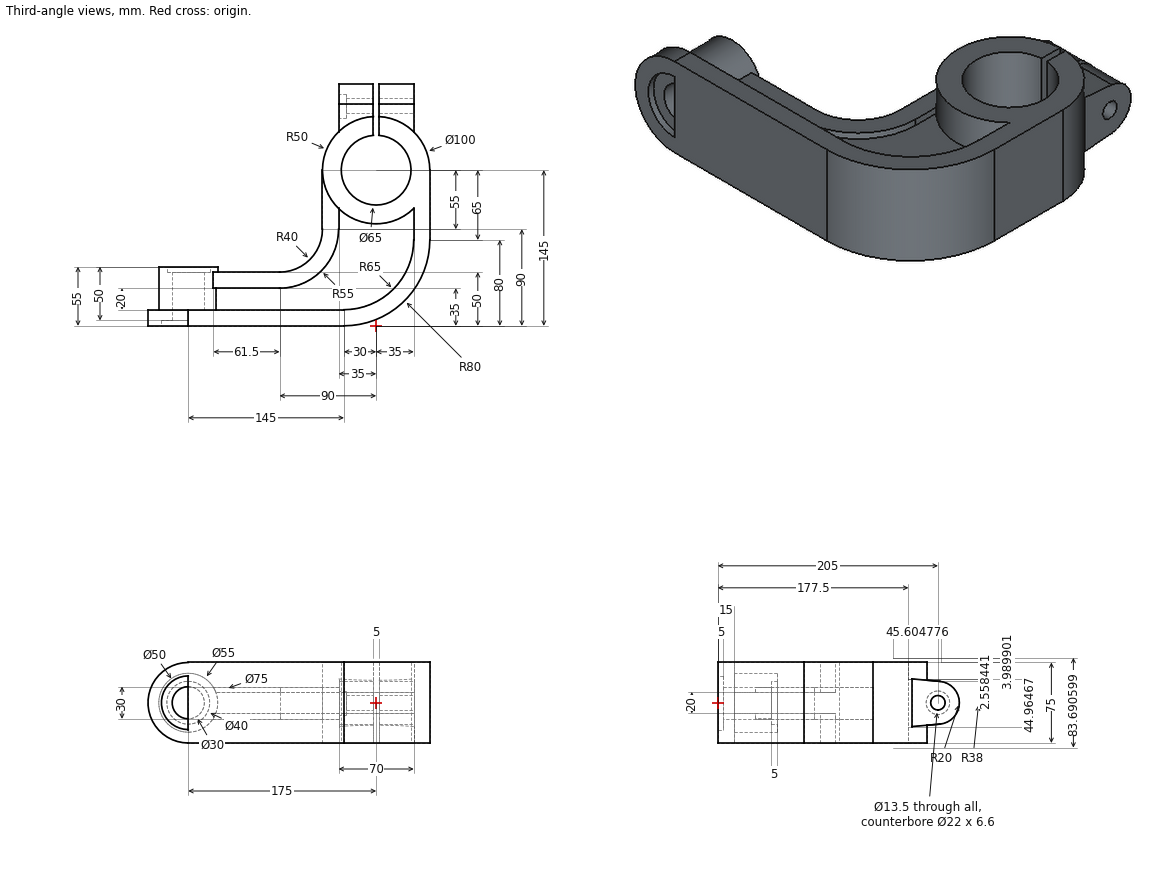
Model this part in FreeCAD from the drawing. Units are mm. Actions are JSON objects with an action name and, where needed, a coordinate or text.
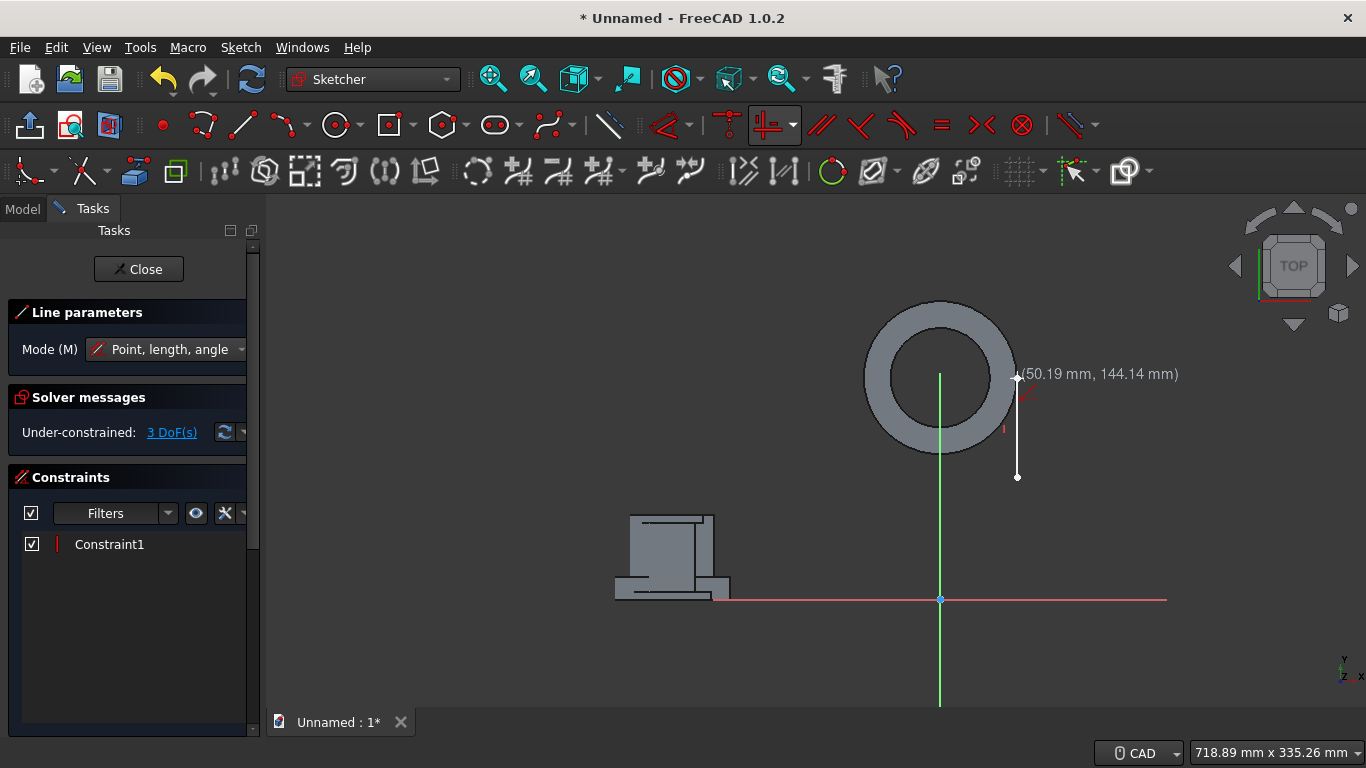
{"action": "left_click", "coordinate": [994, 432]}
{"action": "left_click", "coordinate": [994, 477]}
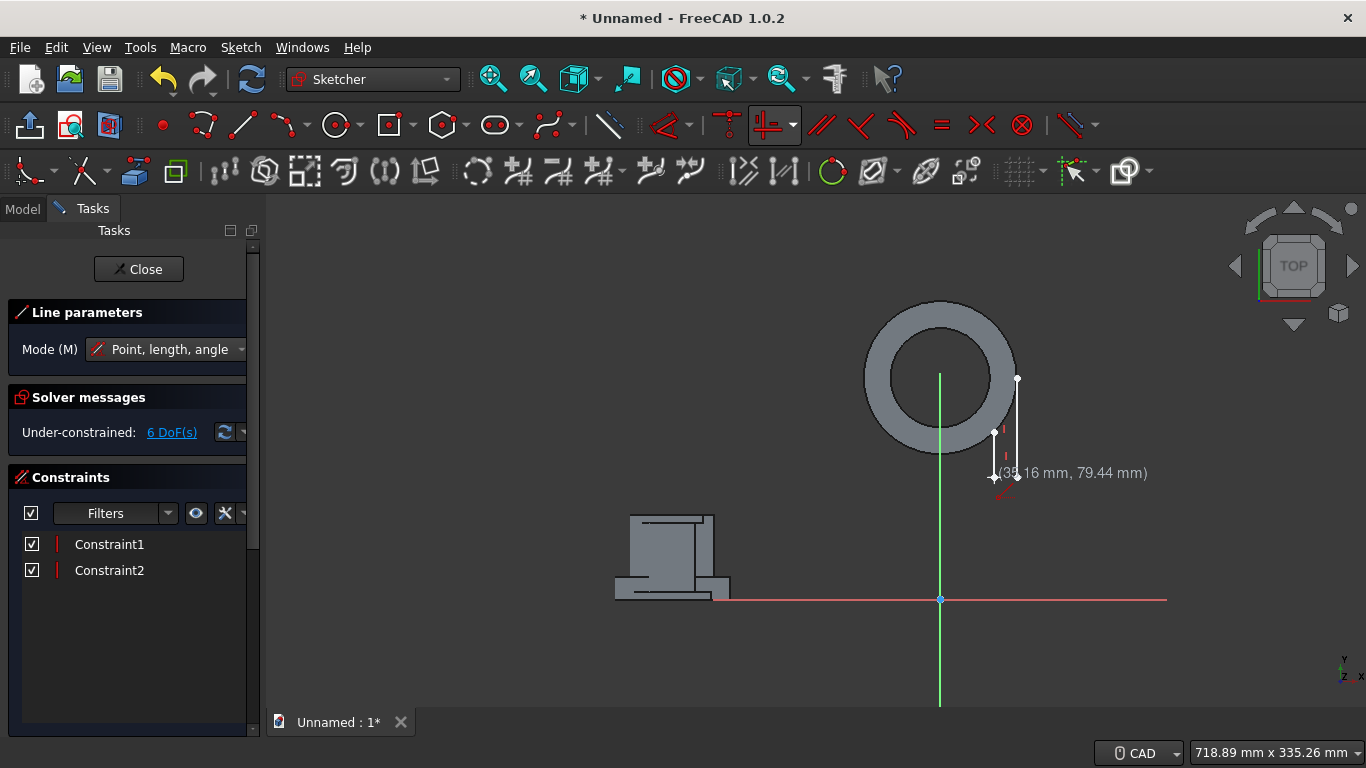
{"action": "key", "text": "g m"}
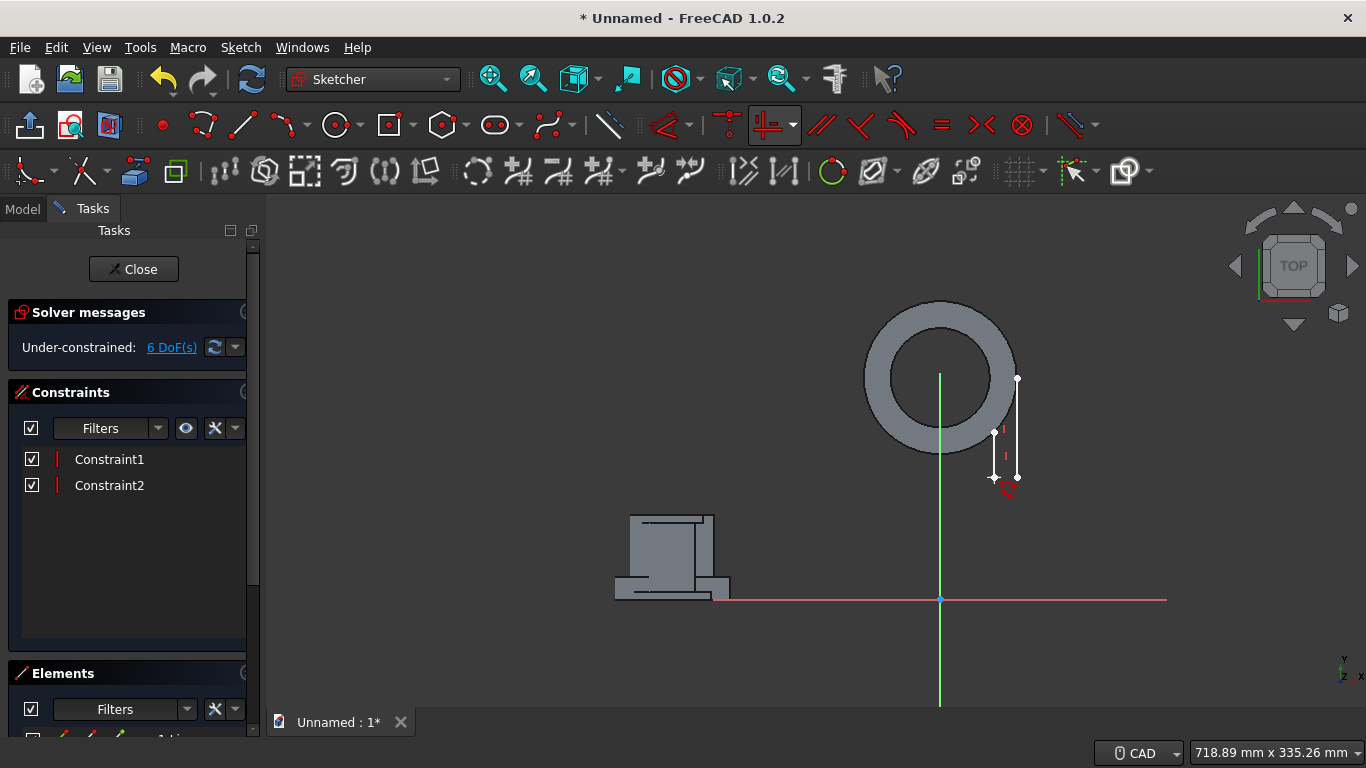
{"action": "left_click", "coordinate": [894, 577]}
{"action": "left_click", "coordinate": [672, 577]}
{"action": "left_click", "coordinate": [672, 600]}
{"action": "left_click", "coordinate": [894, 591]}
{"action": "right_click", "coordinate": [894, 591]}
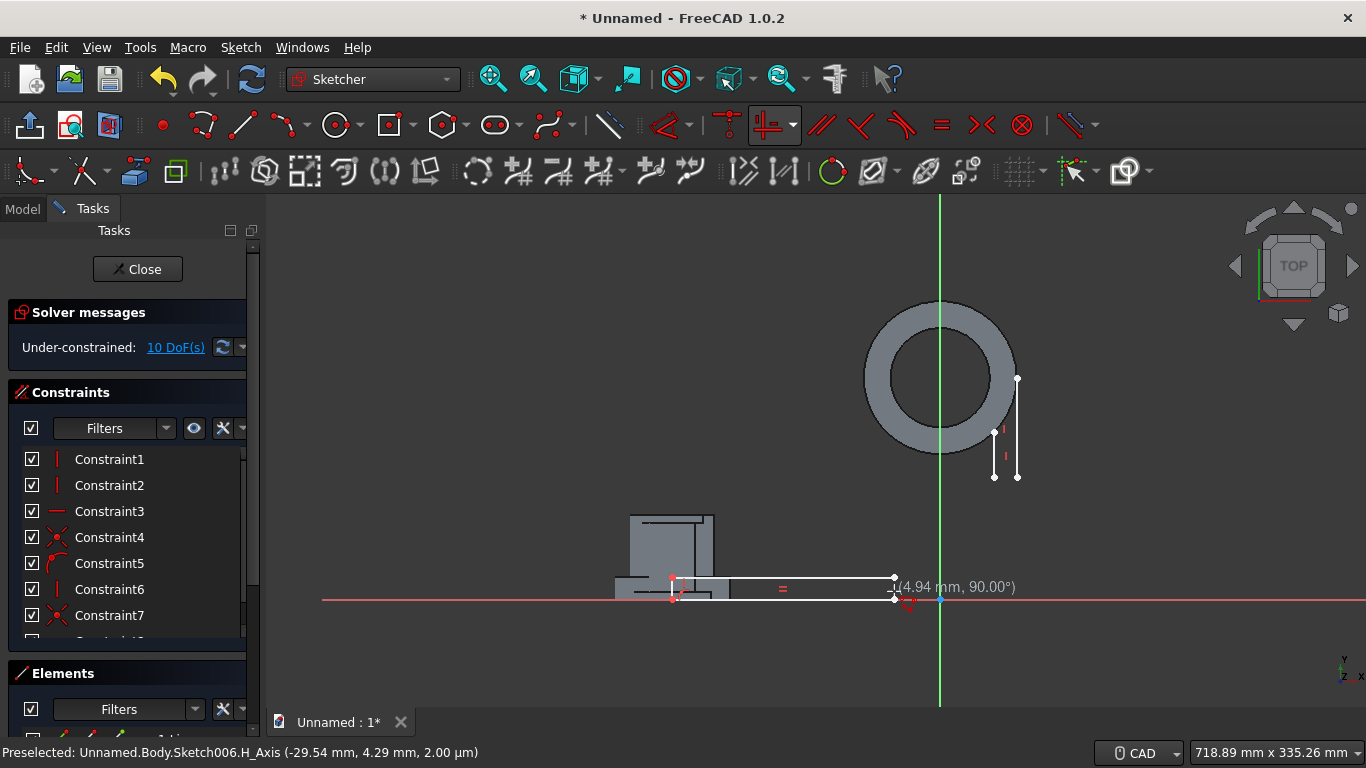
{"action": "key", "text": "g 3 a"}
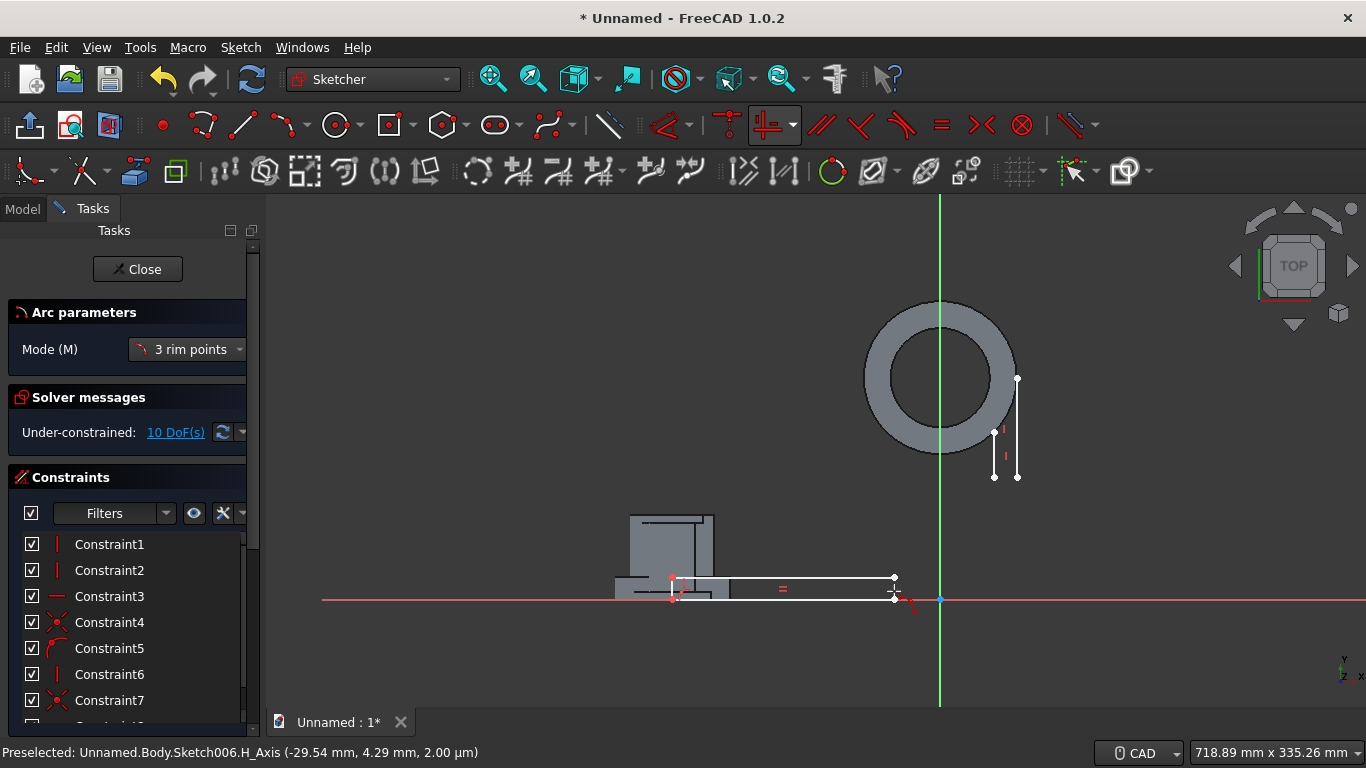
{"action": "left_click", "coordinate": [1017, 379]}
{"action": "left_click", "coordinate": [994, 433]}
{"action": "left_click", "coordinate": [870, 348]}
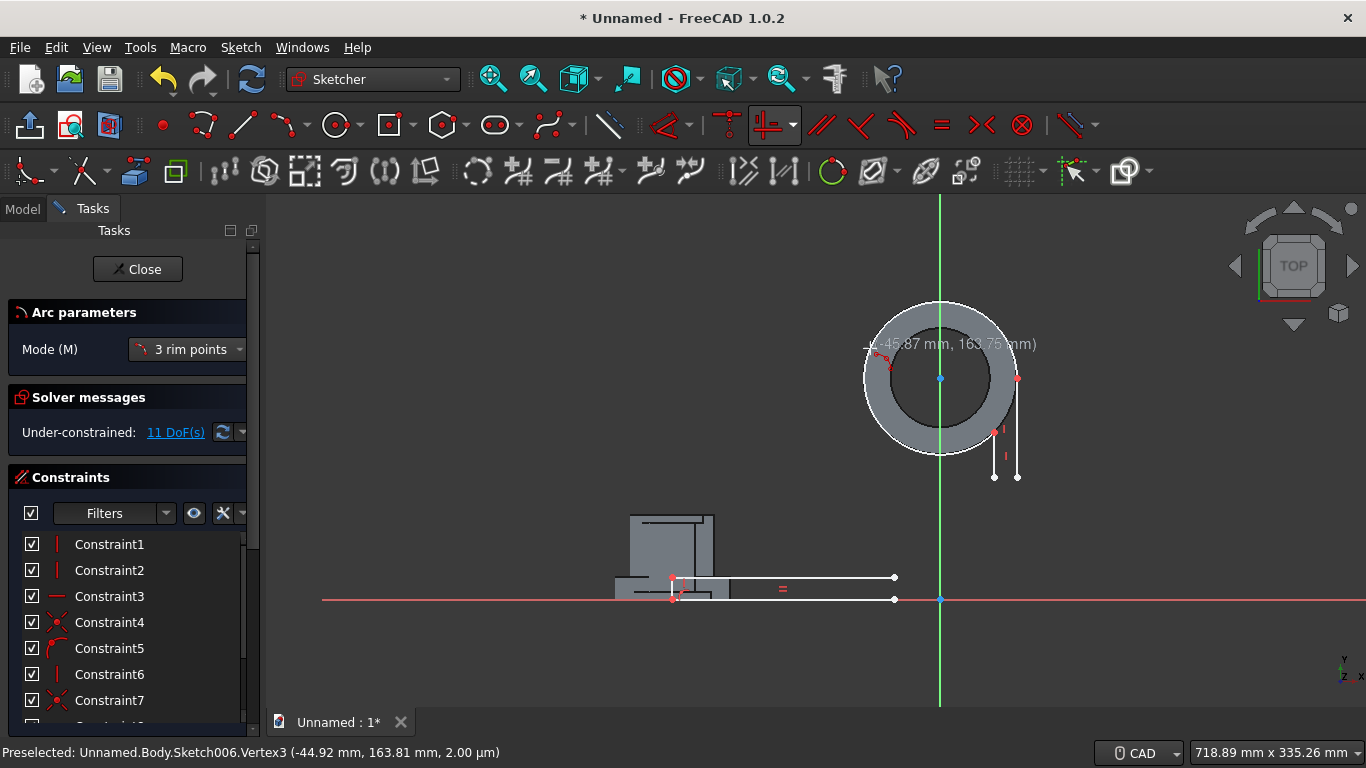
{"action": "left_click", "coordinate": [994, 478]}
{"action": "left_click", "coordinate": [894, 578]}
{"action": "left_click", "coordinate": [965, 547]}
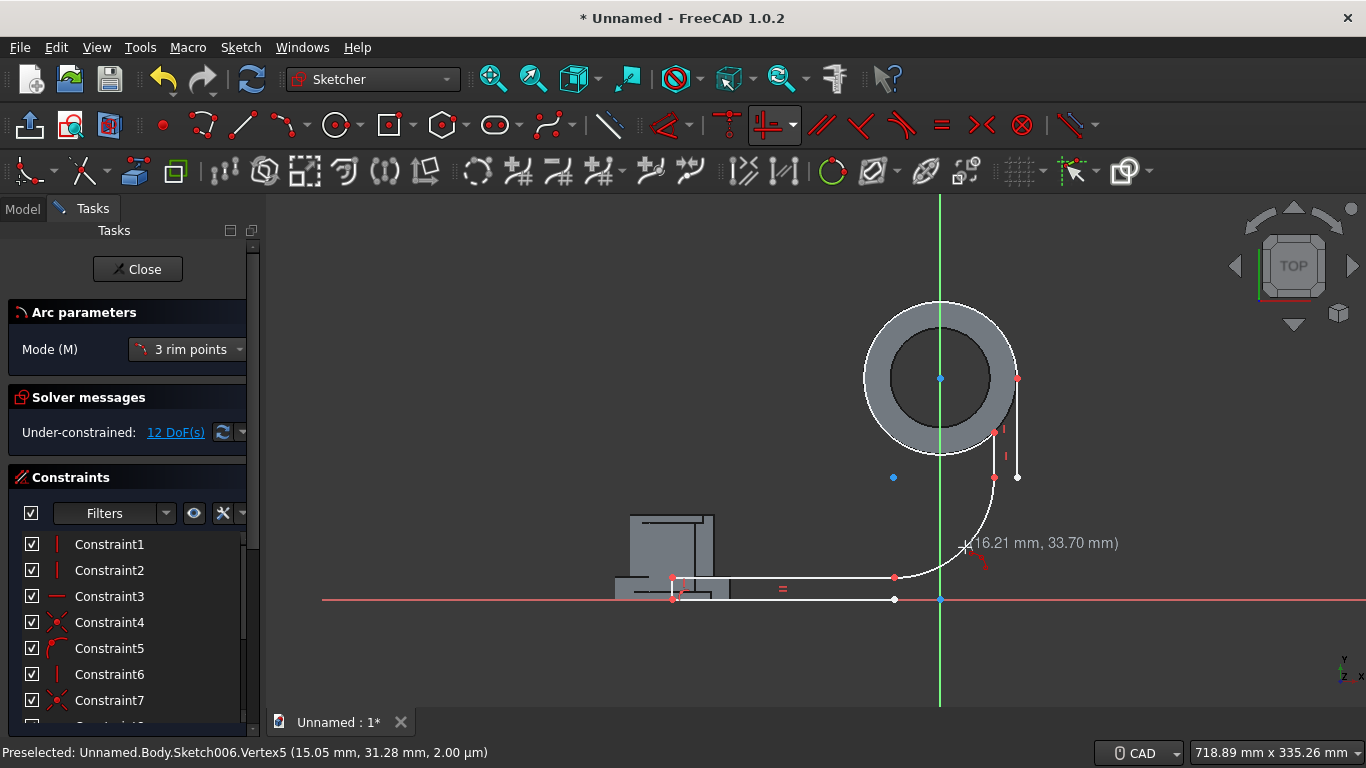
{"action": "left_click", "coordinate": [894, 600]}
{"action": "left_click", "coordinate": [1017, 478]}
{"action": "left_click", "coordinate": [981, 564]}
{"action": "key", "text": "Escape"}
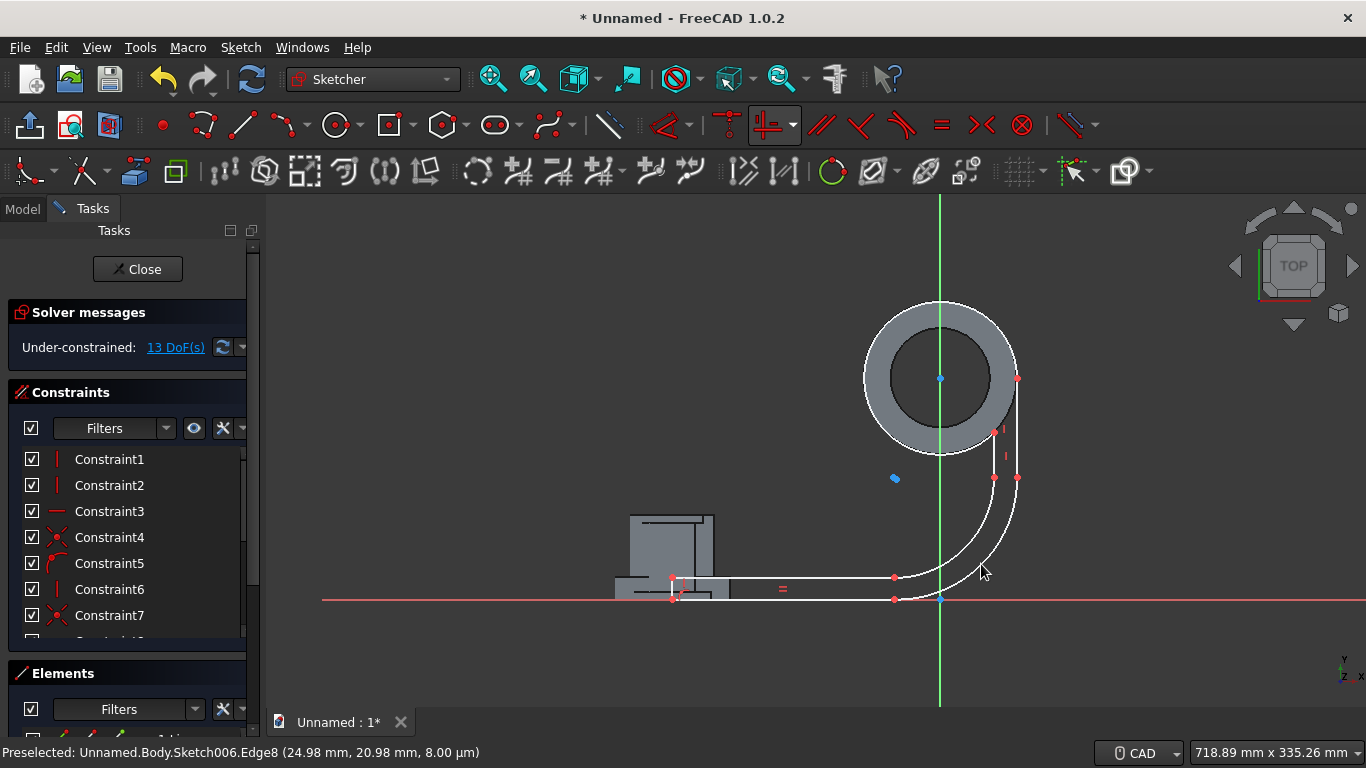
{"action": "left_click", "coordinate": [939, 567]}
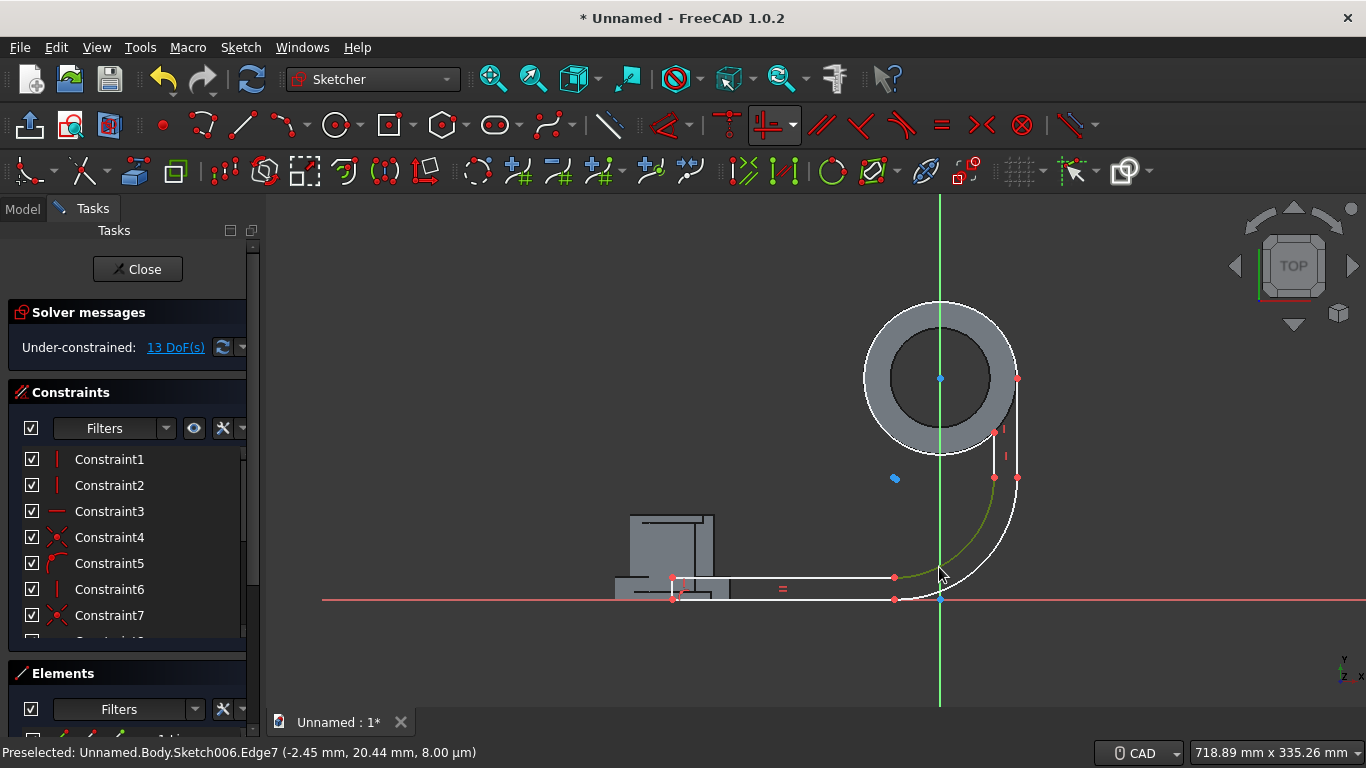
{"action": "scroll", "coordinate": [950, 587], "scroll_direction": "up", "scroll_amount": 2}